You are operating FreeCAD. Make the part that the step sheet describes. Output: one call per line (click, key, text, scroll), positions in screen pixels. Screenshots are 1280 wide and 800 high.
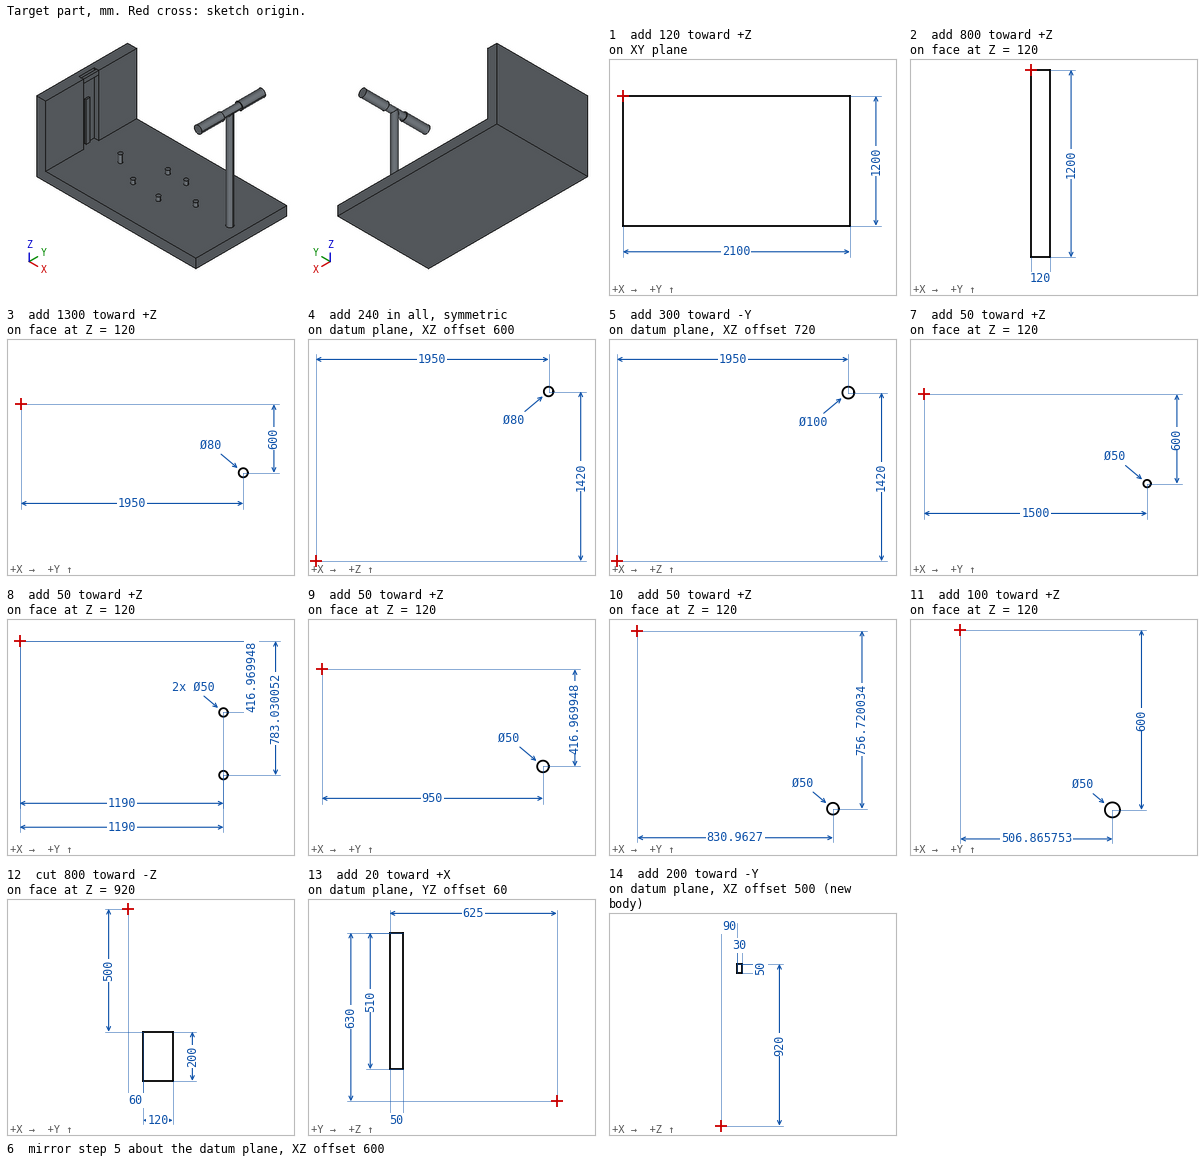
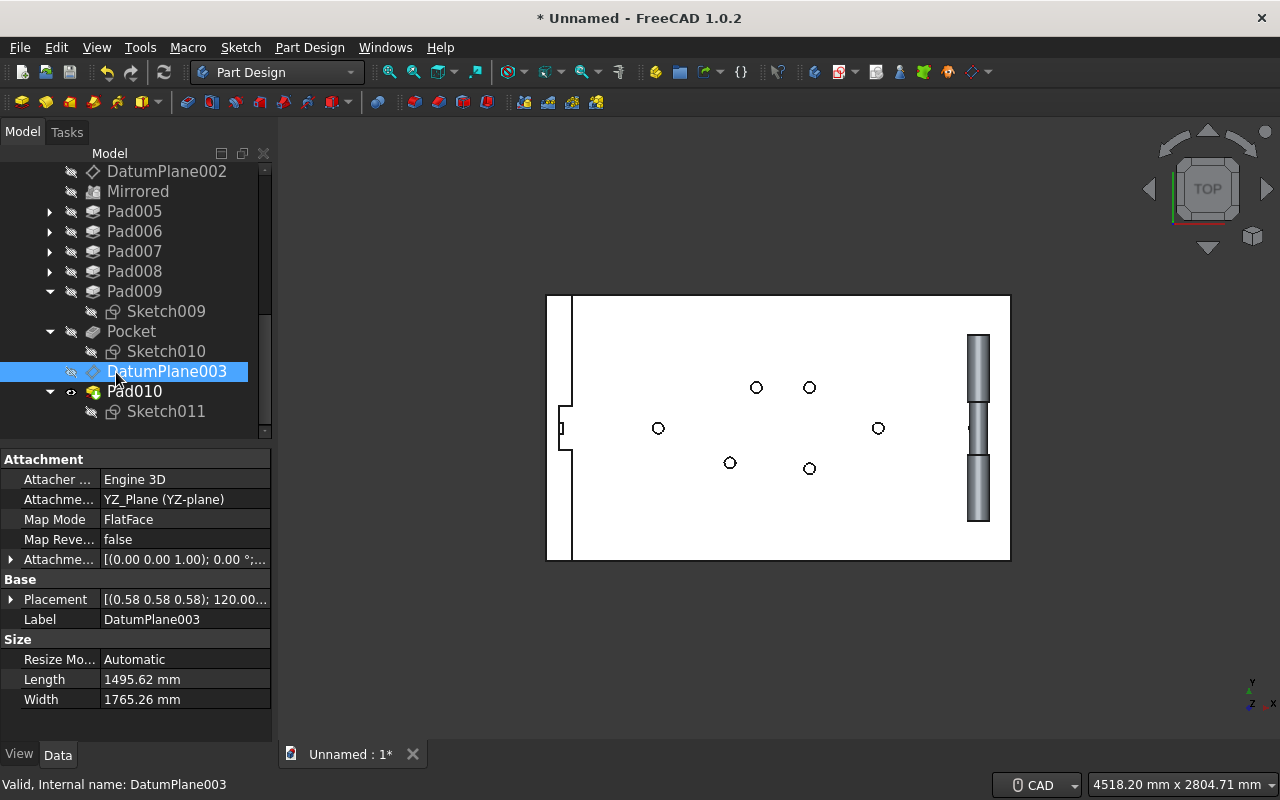
click(318, 699)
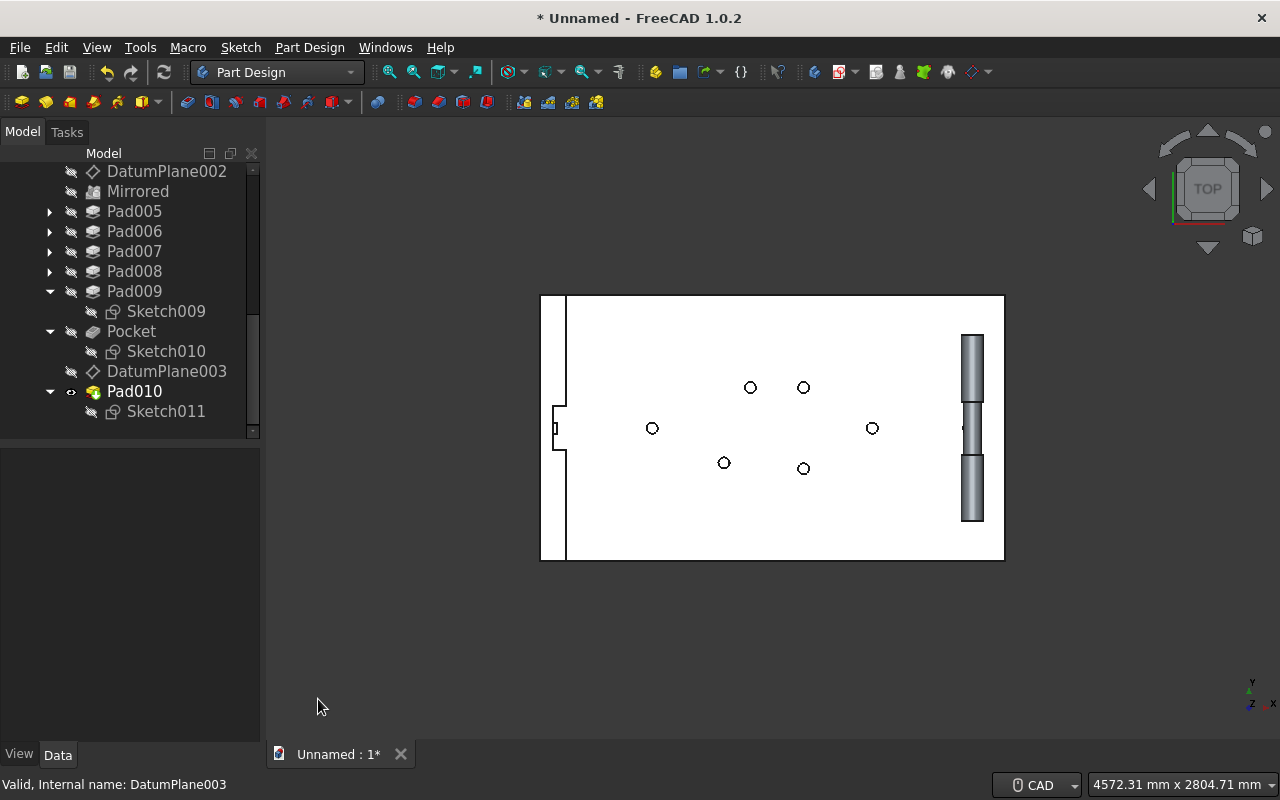
click(816, 72)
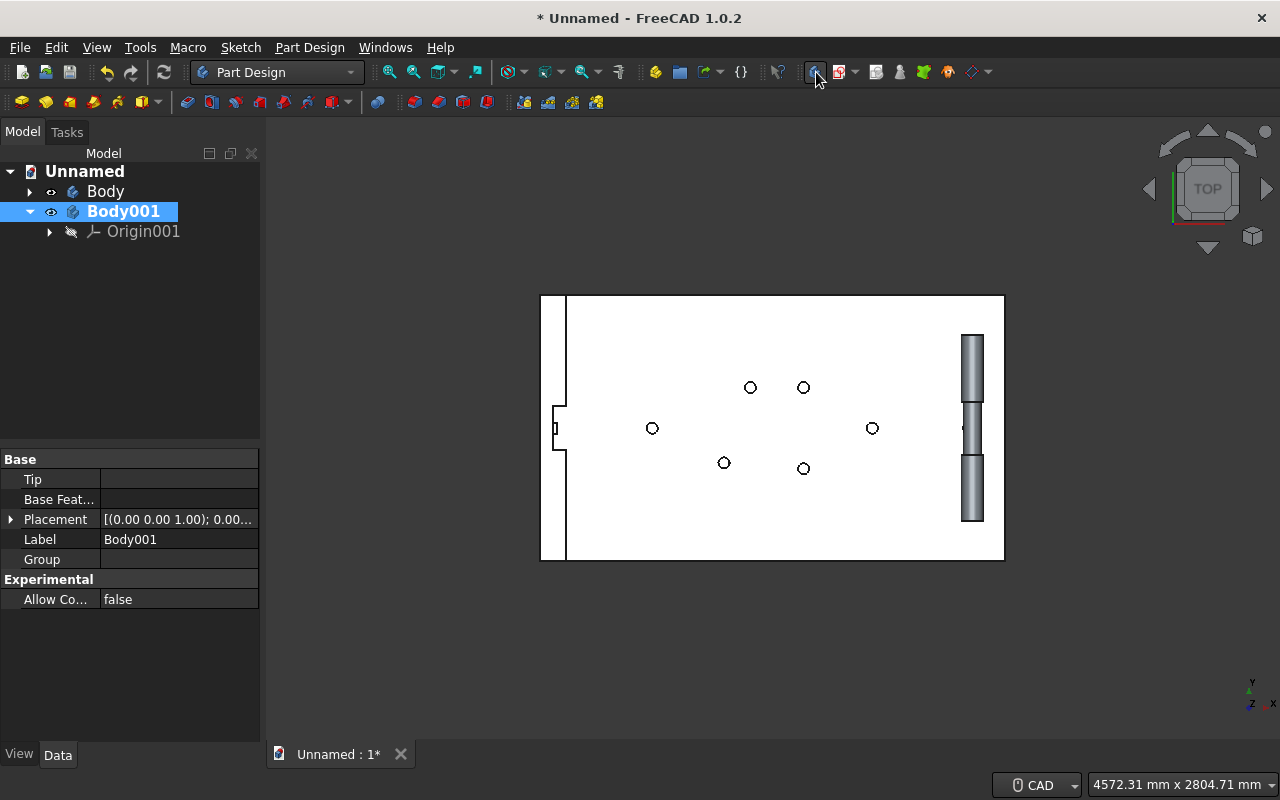
click(50, 232)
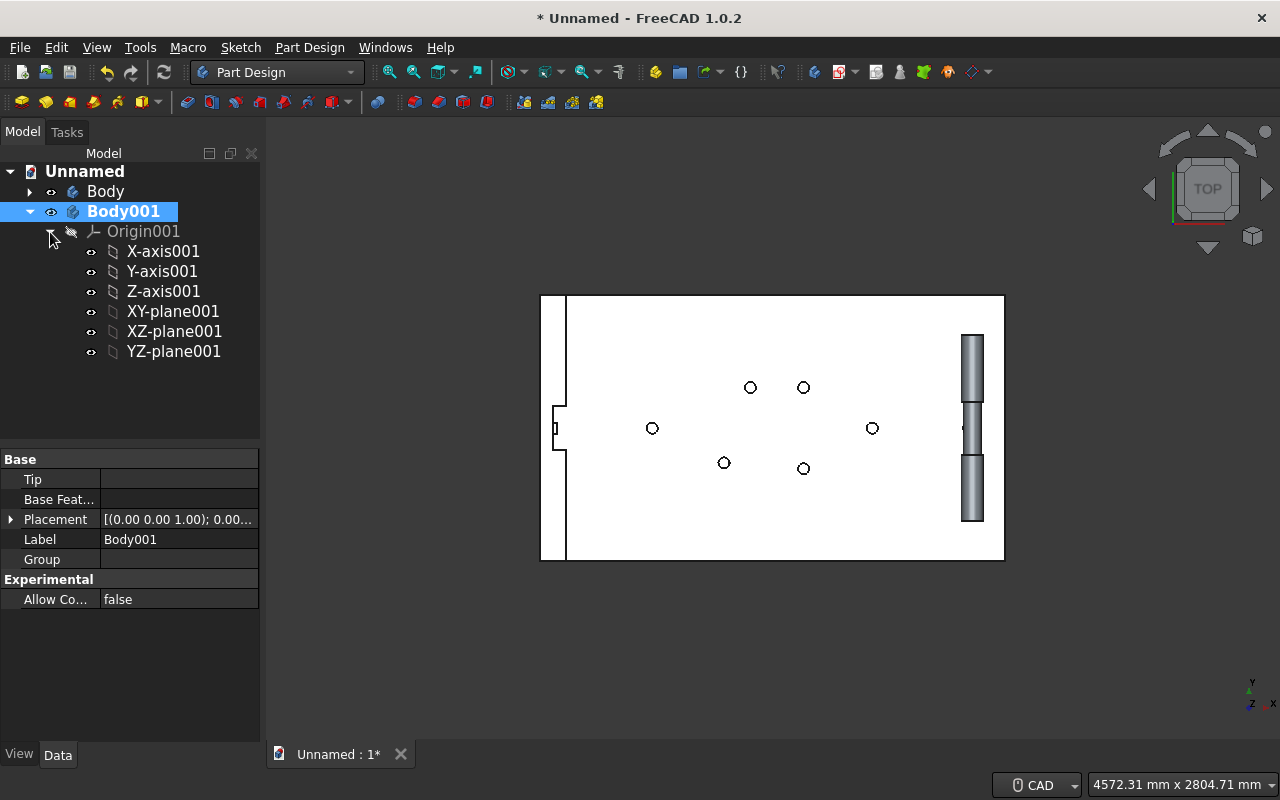
click(136, 332)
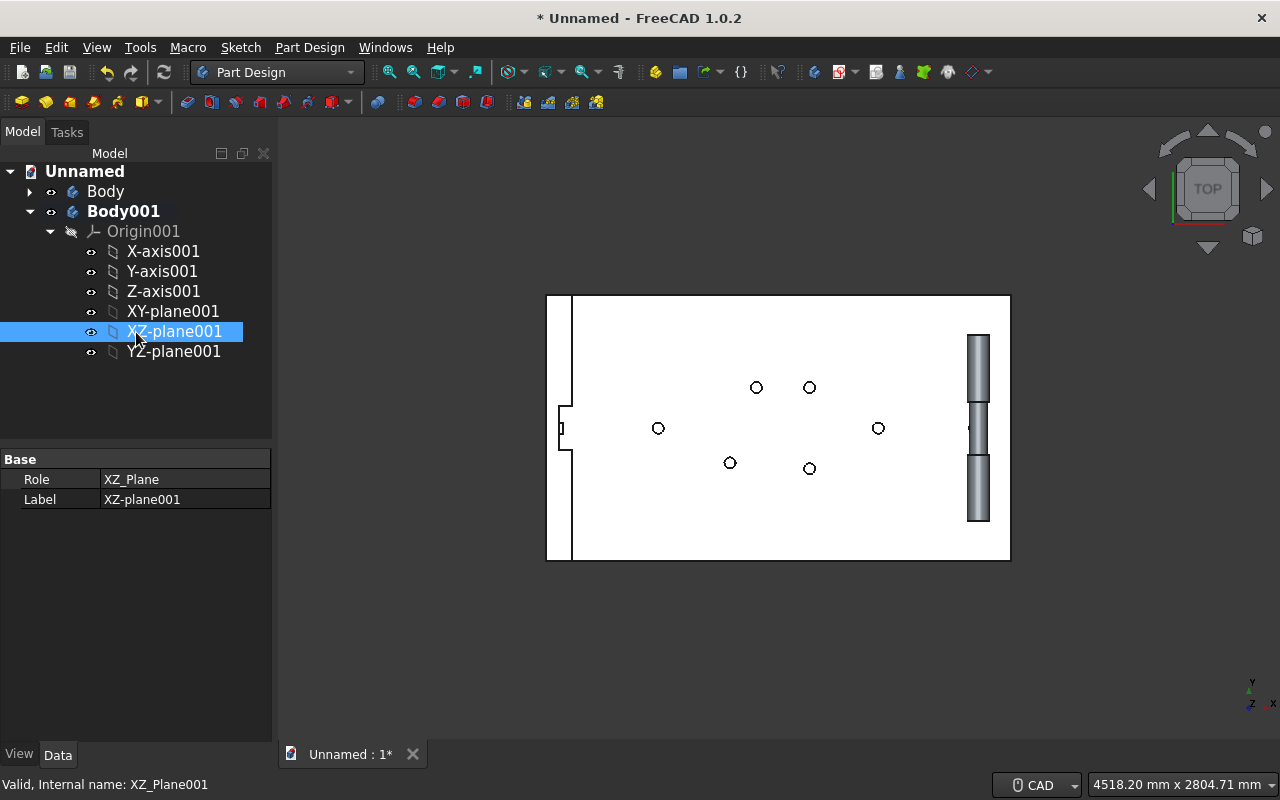
click(972, 72)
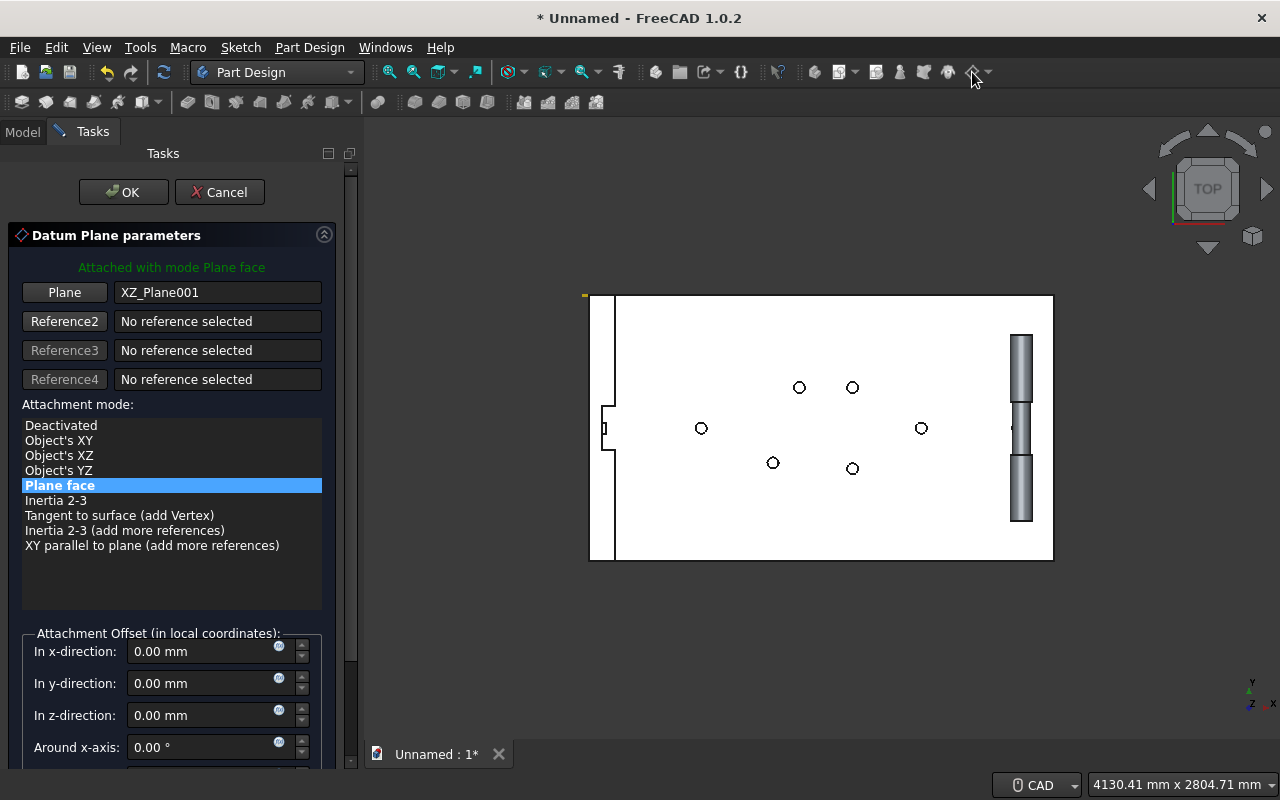
triple_click(210, 715)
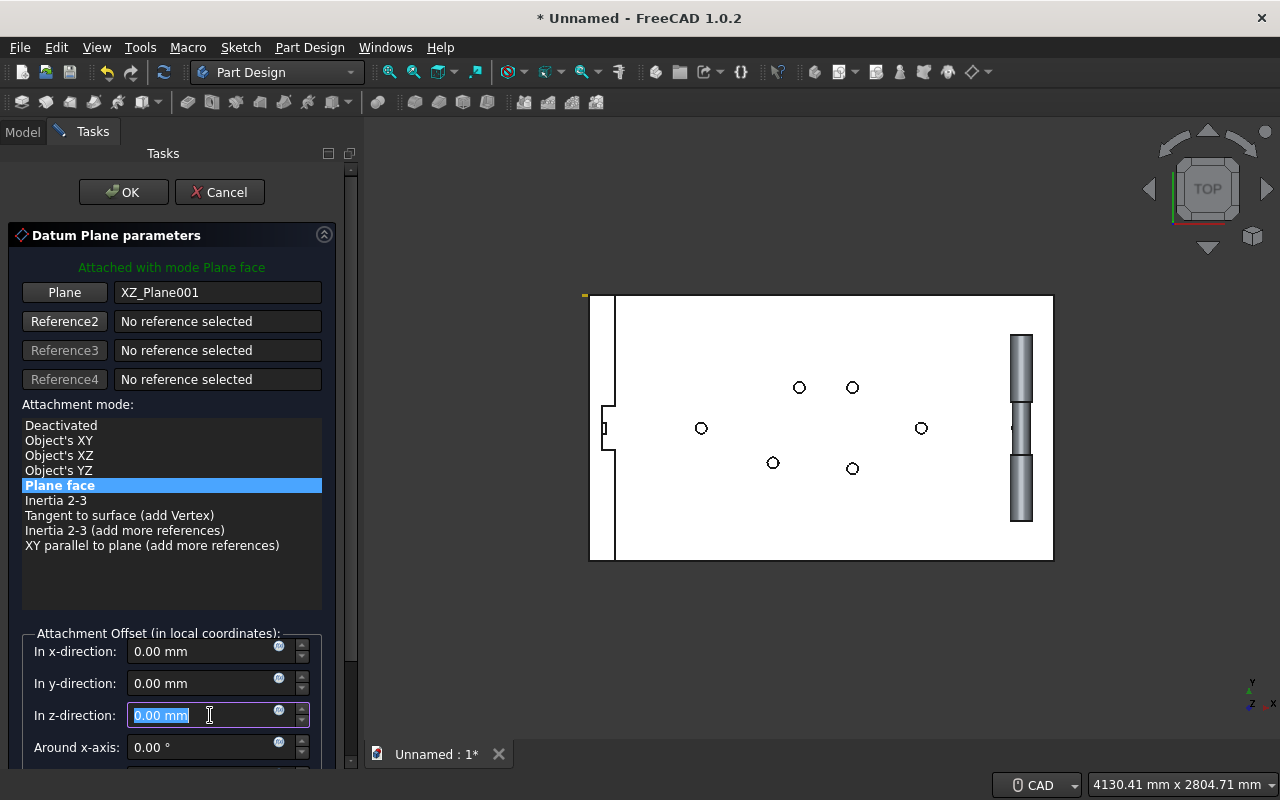
text(500)
key(Tab)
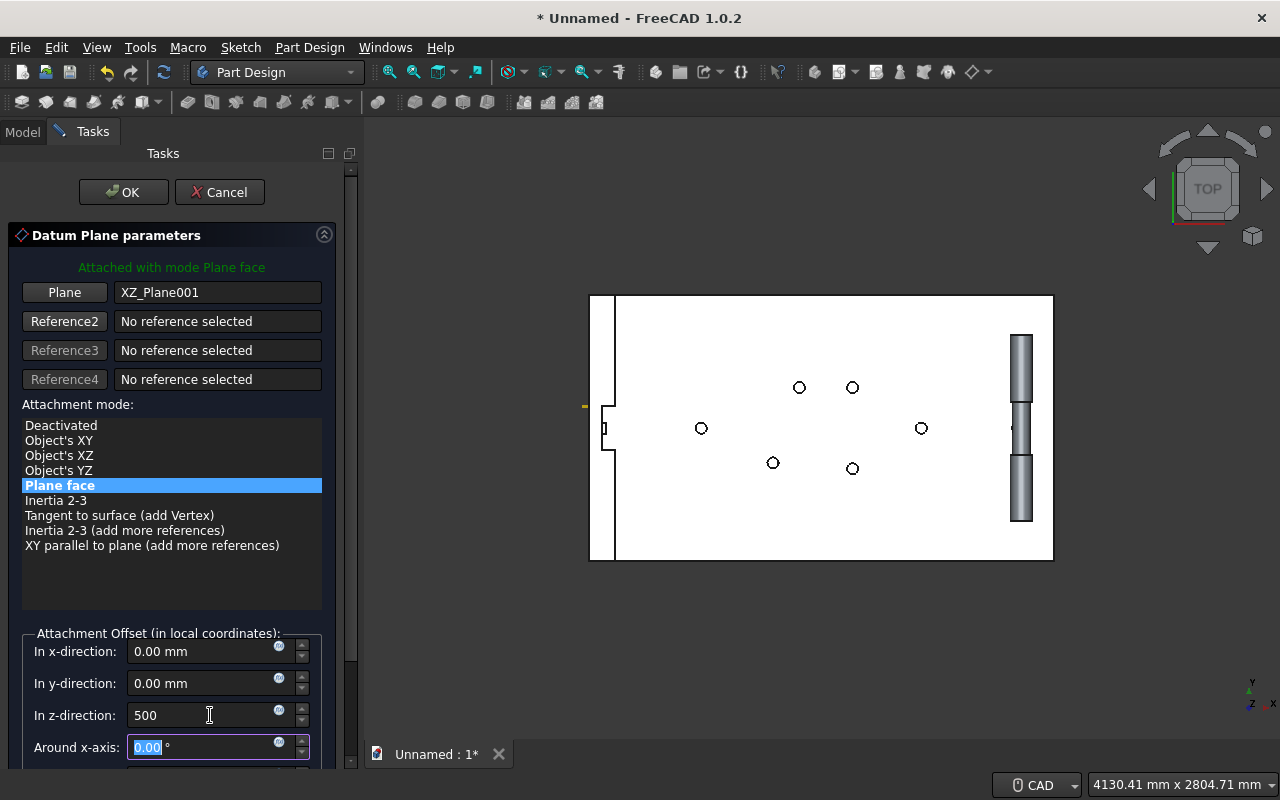
click(124, 192)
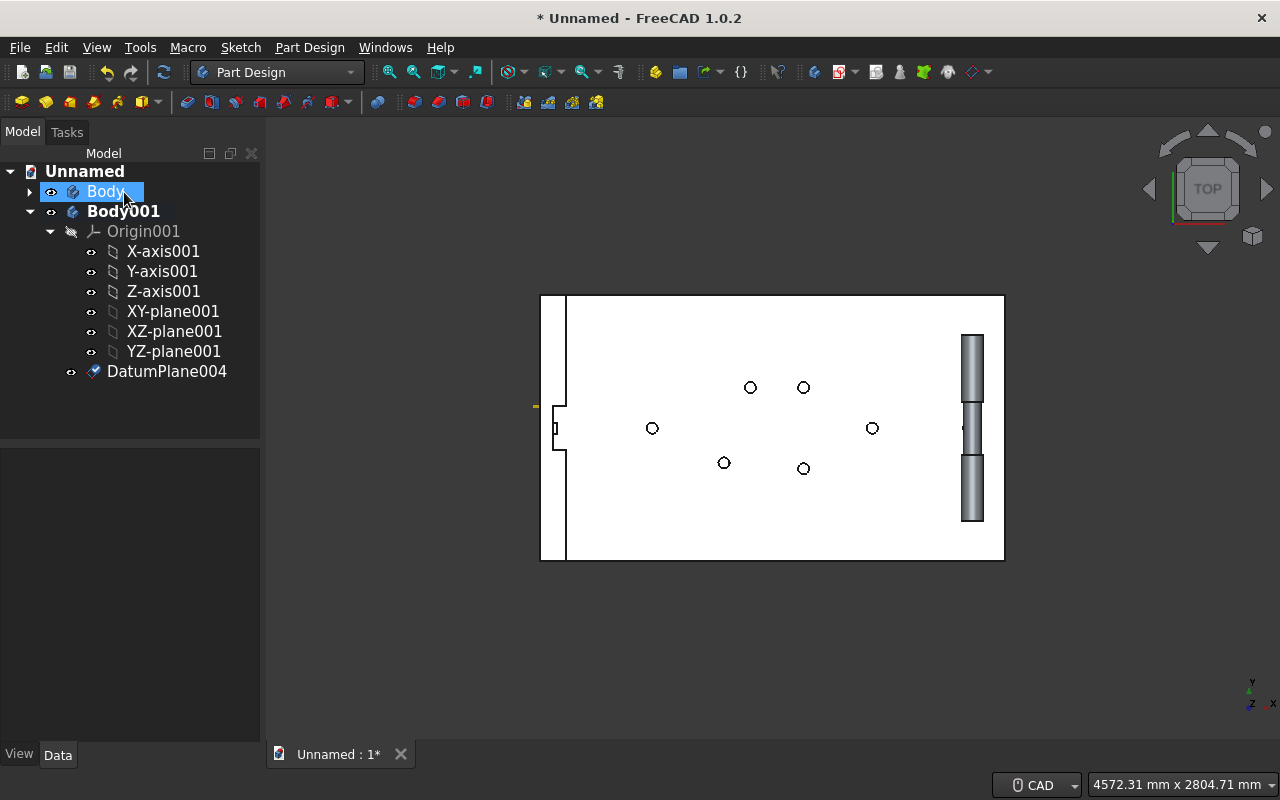
click(116, 372)